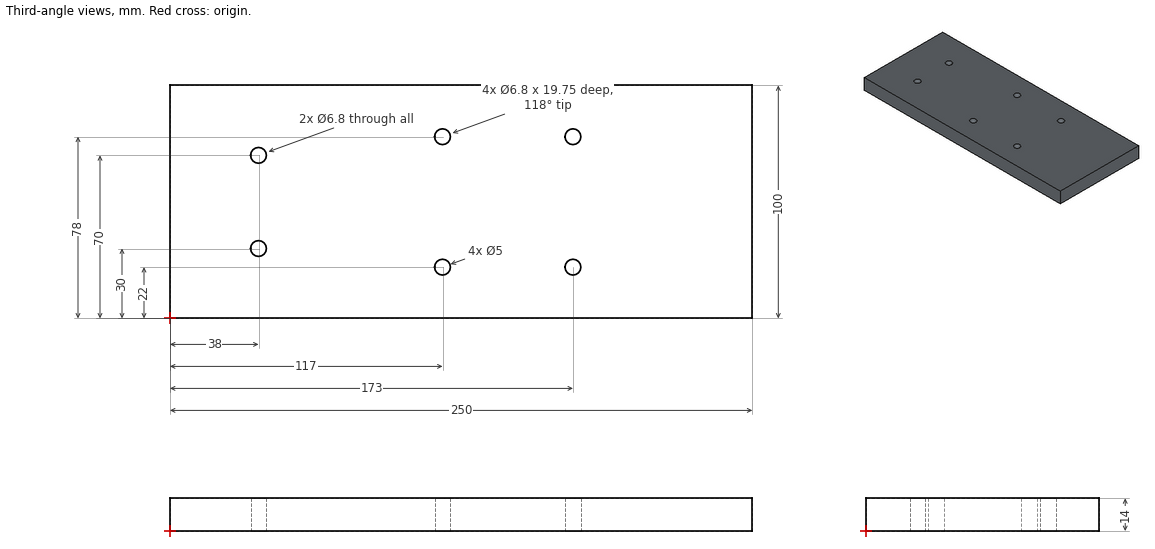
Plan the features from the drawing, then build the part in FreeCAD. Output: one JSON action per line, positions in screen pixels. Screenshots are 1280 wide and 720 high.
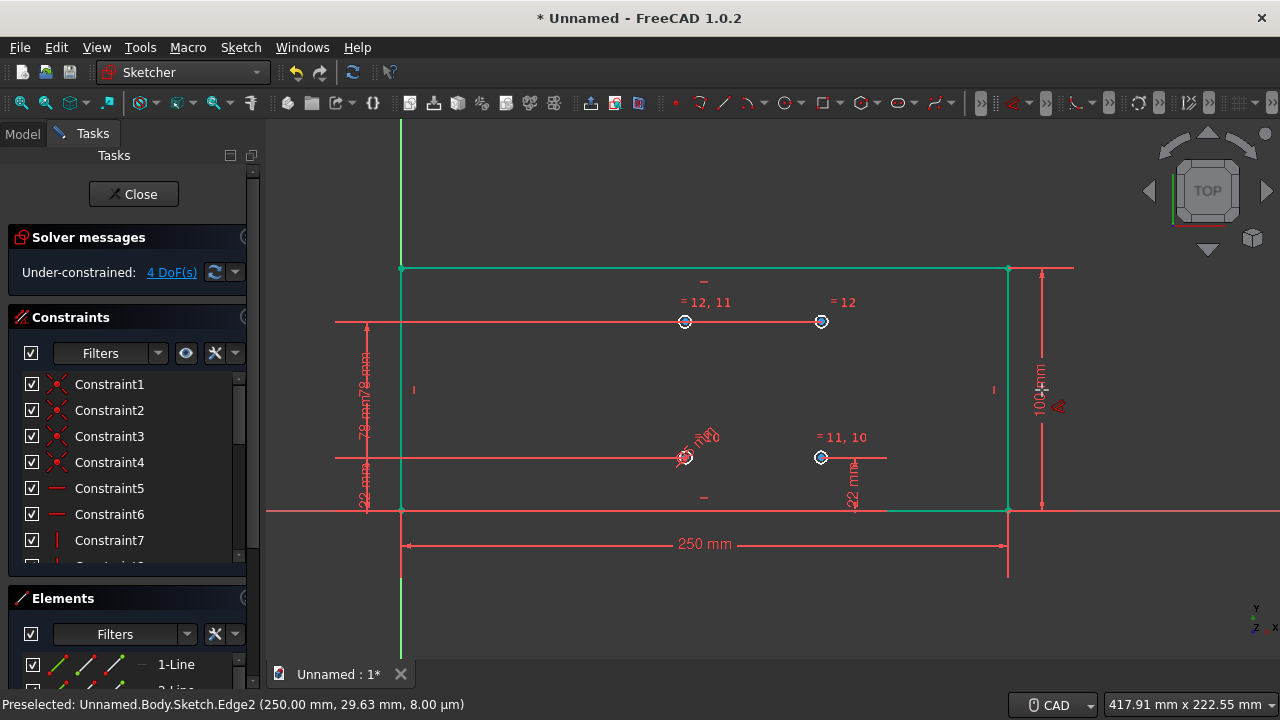
{"action": "left_click", "coordinate": [686, 458]}
{"action": "left_click", "coordinate": [544, 545]}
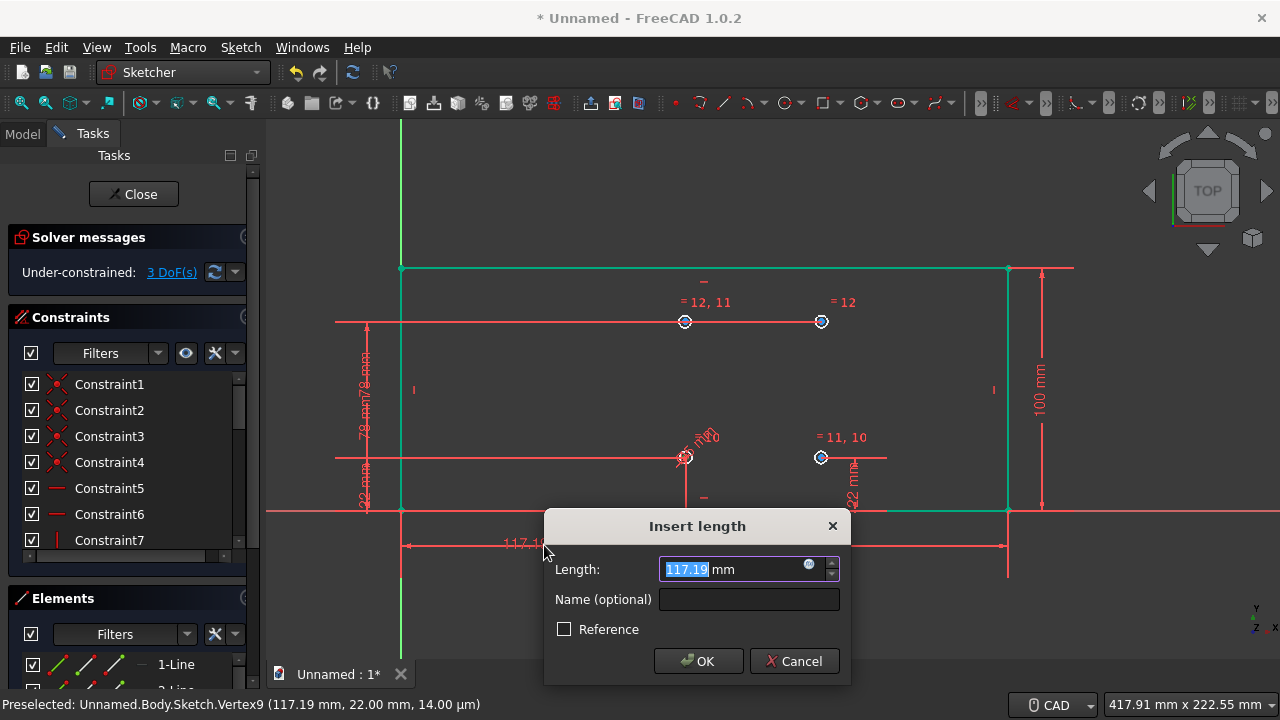
{"action": "type", "text": "117"}
{"action": "key", "text": "Return"}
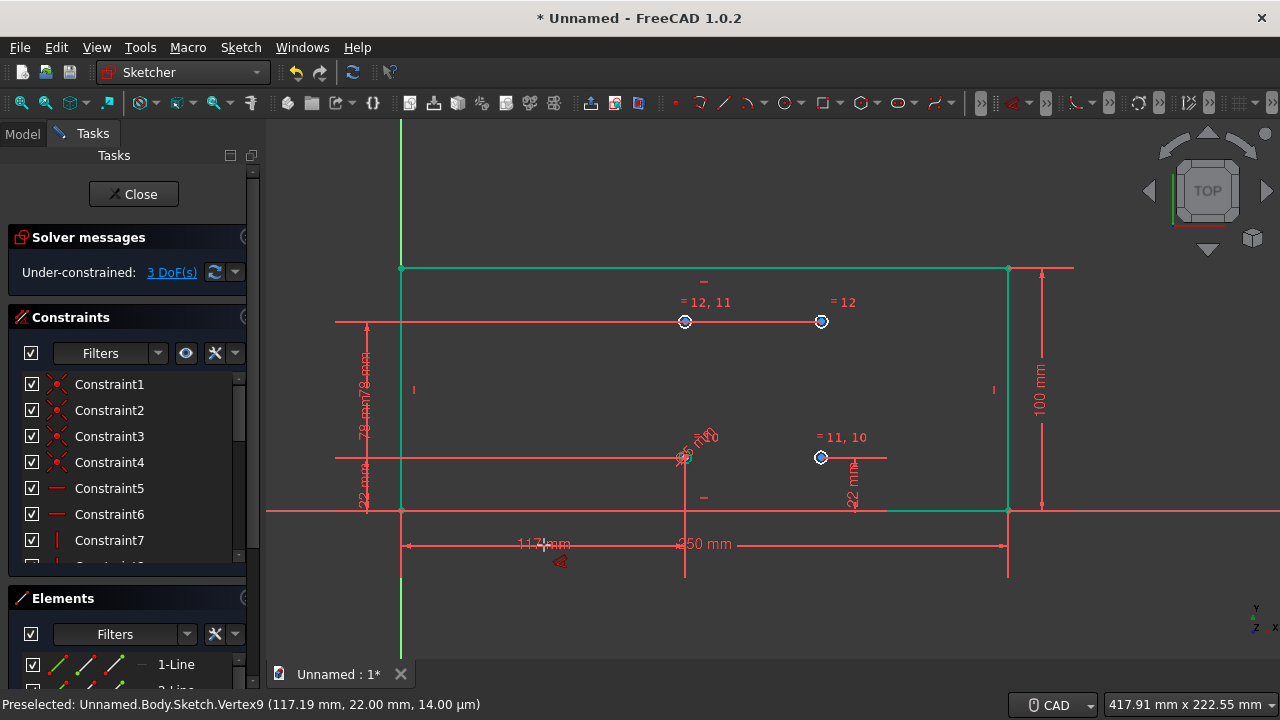
{"action": "left_click", "coordinate": [821, 458]}
{"action": "left_click", "coordinate": [464, 545]}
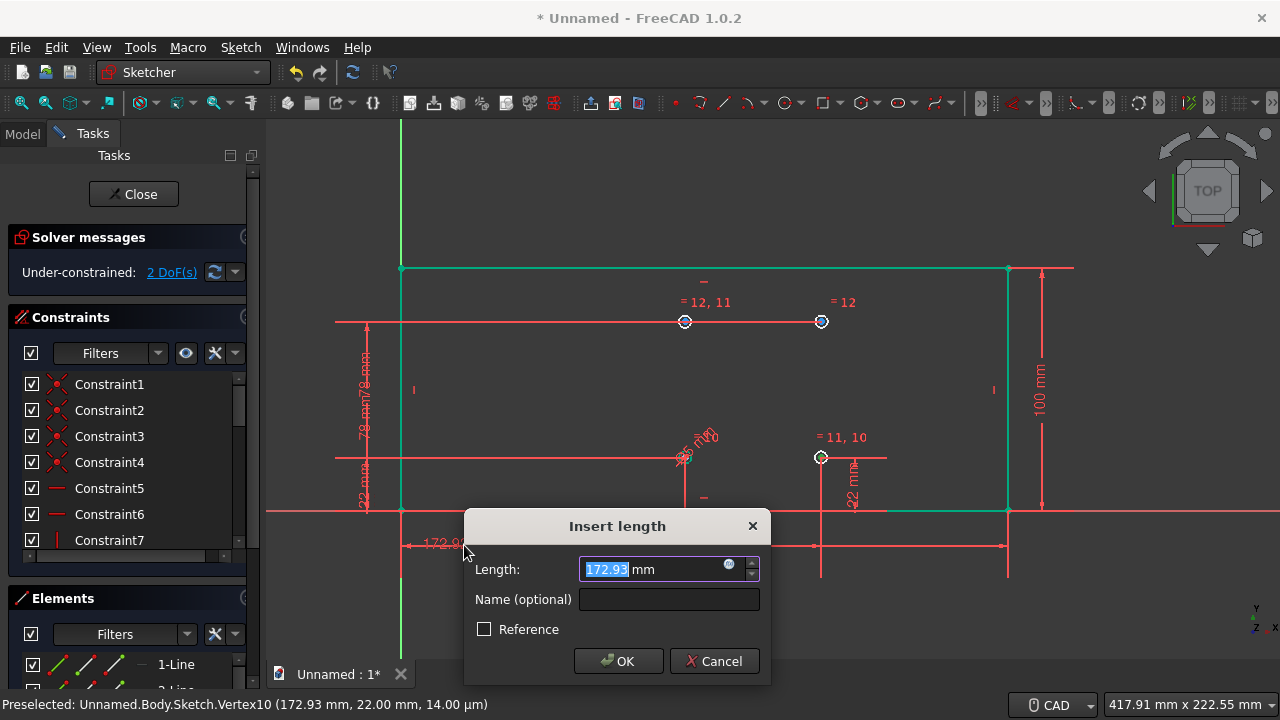
{"action": "type", "text": "173"}
{"action": "key", "text": "Return"}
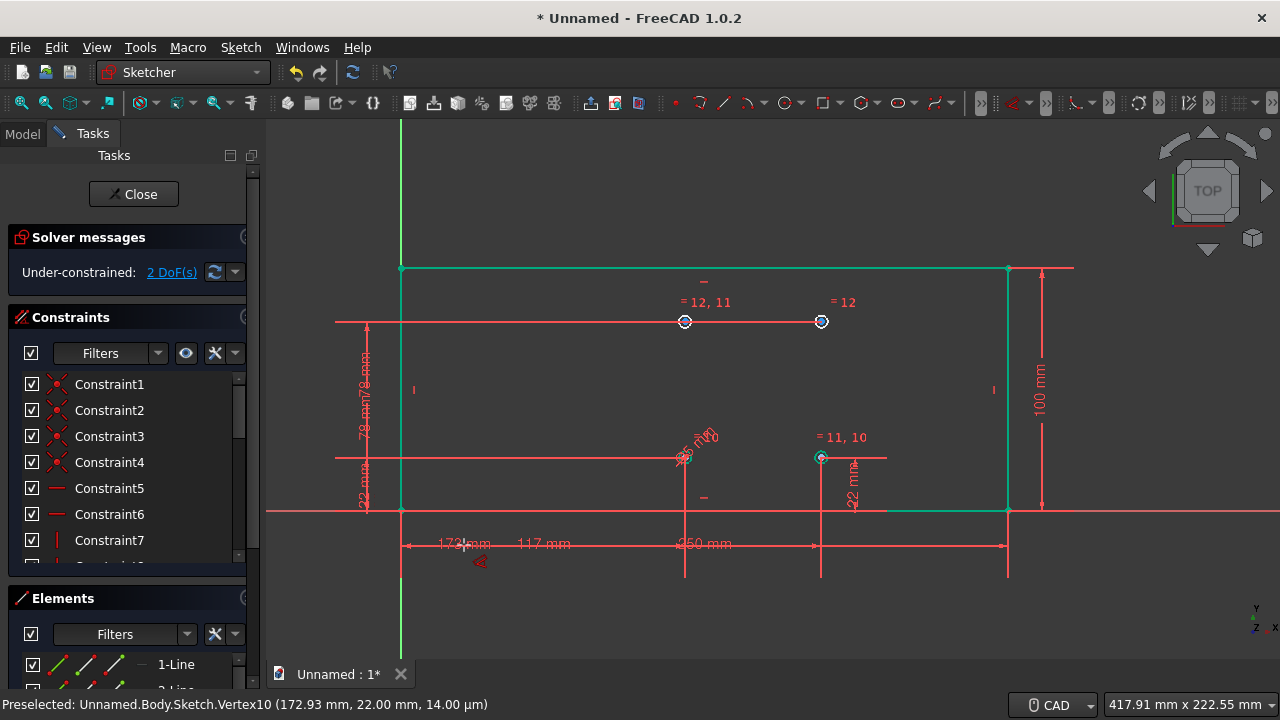
{"action": "left_click", "coordinate": [685, 322]}
{"action": "left_click", "coordinate": [543, 288]}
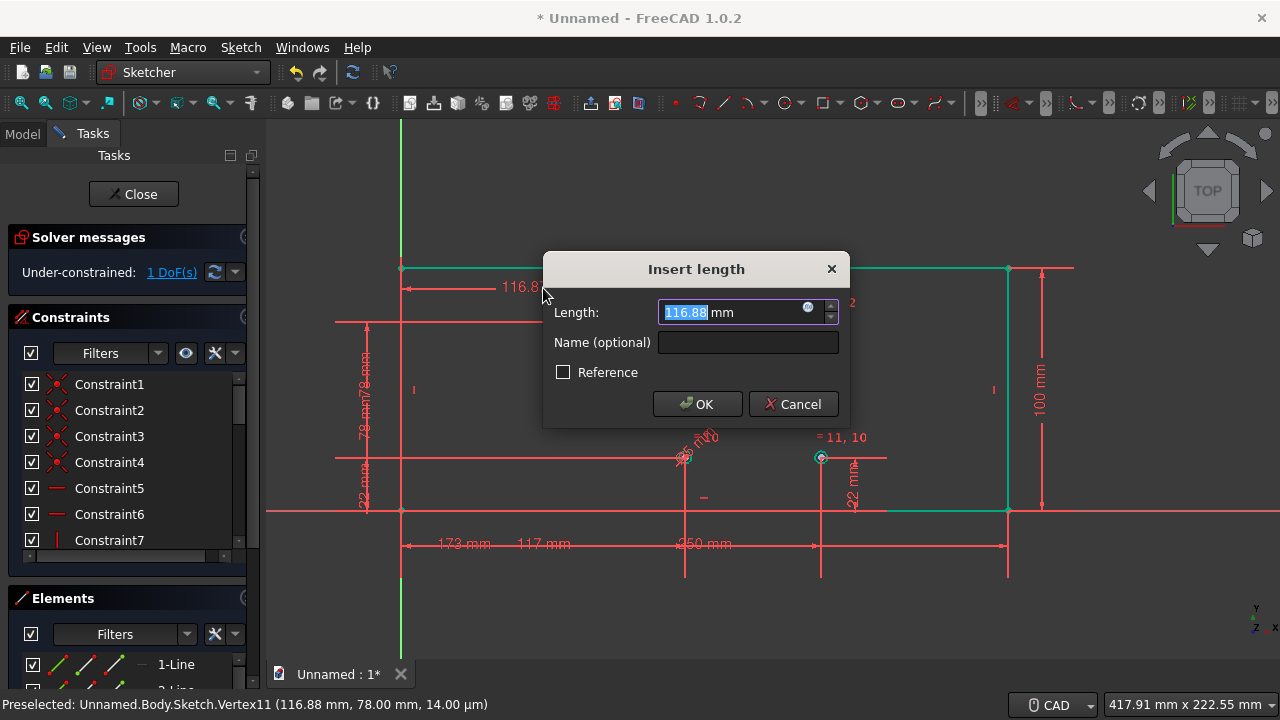
{"action": "type", "text": "117"}
{"action": "key", "text": "Return"}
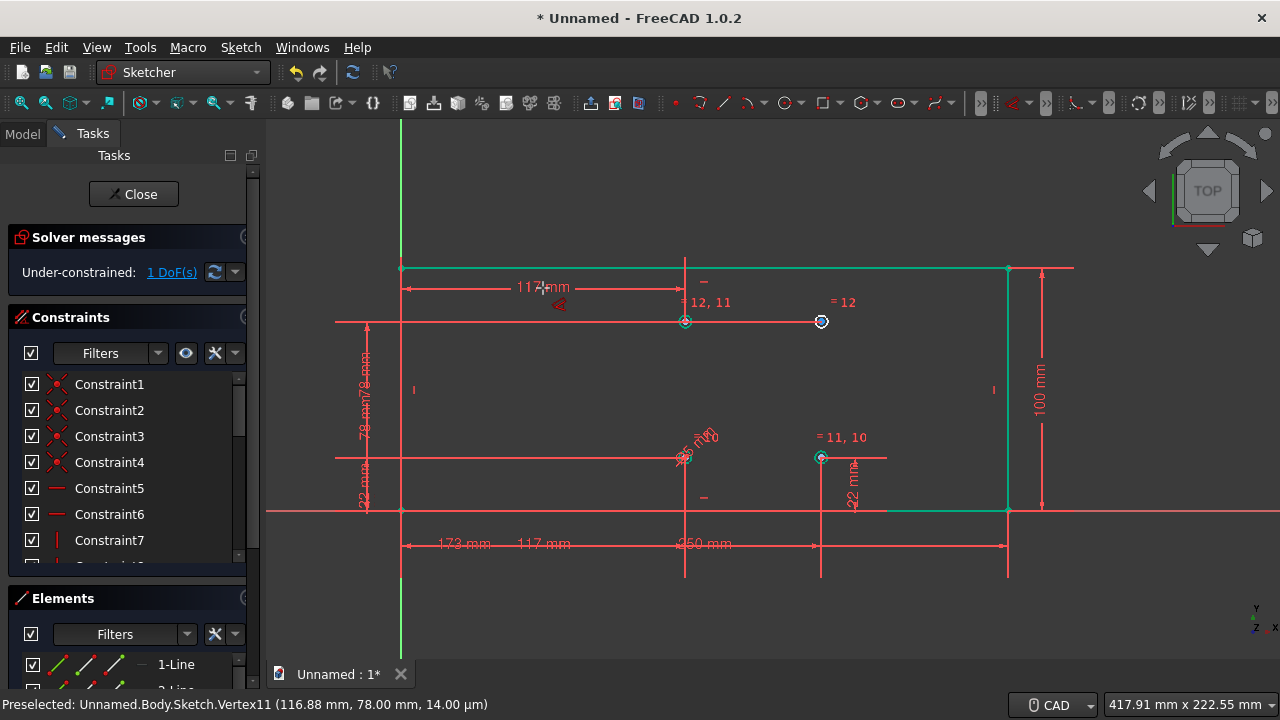
{"action": "left_click", "coordinate": [822, 322]}
{"action": "left_click", "coordinate": [708, 288]}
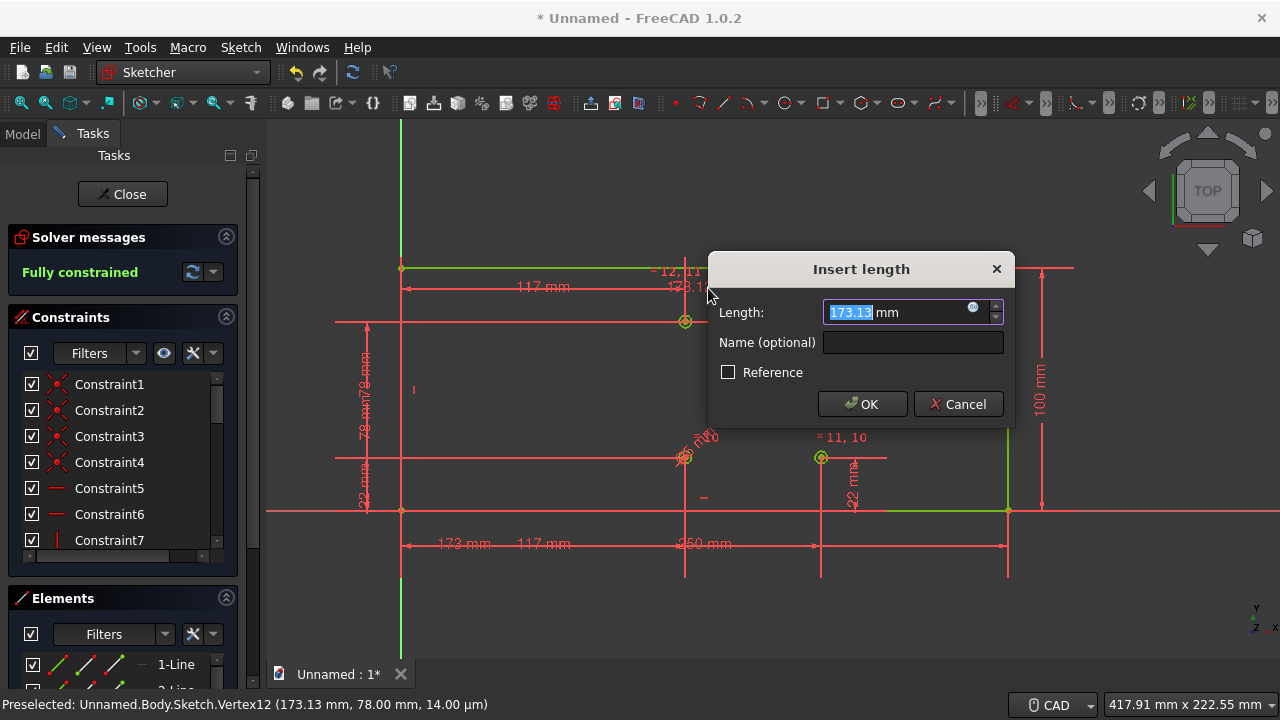
{"action": "type", "text": "173"}
{"action": "key", "text": "Return"}
{"action": "key", "text": "Escape"}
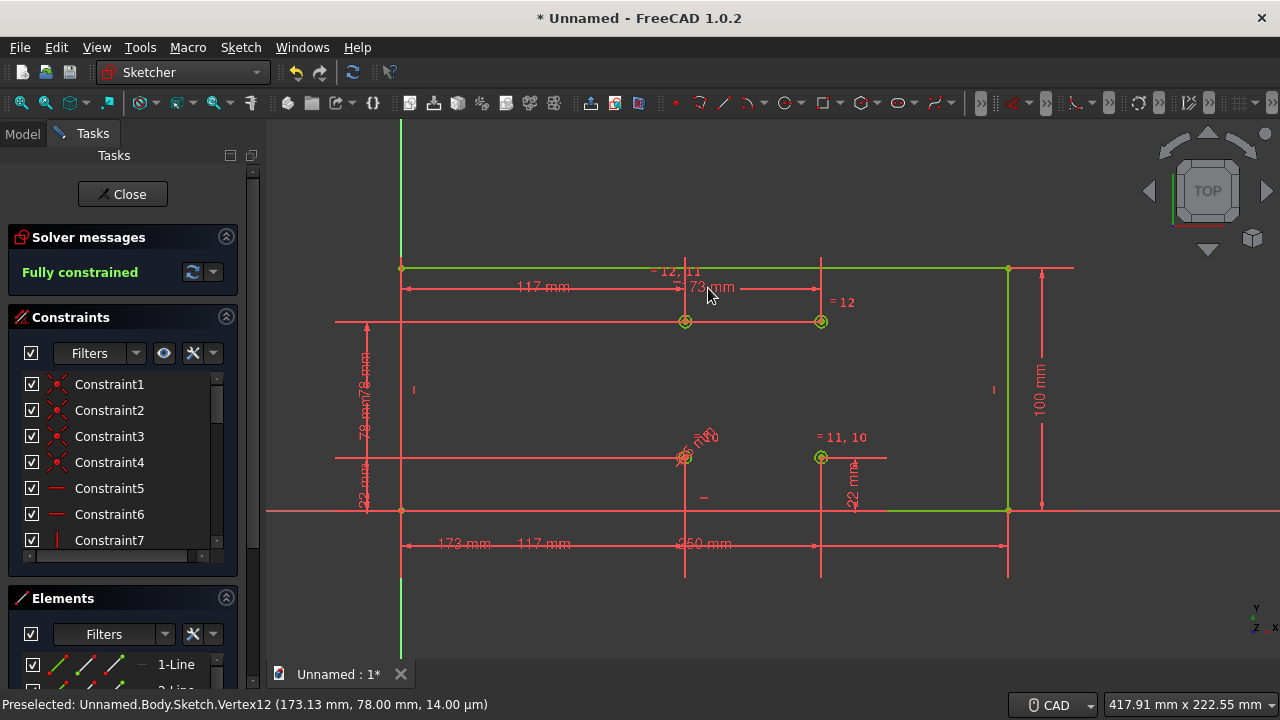
{"action": "left_click", "coordinate": [123, 194]}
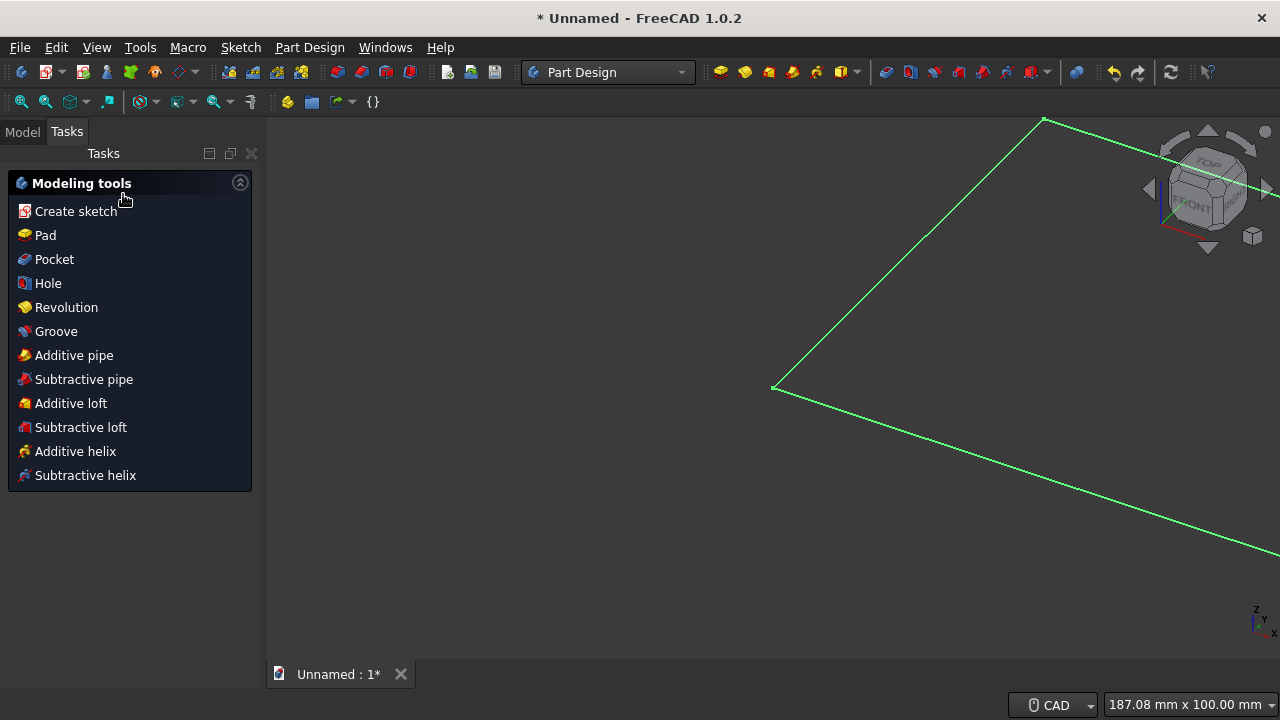
{"action": "left_click", "coordinate": [722, 72]}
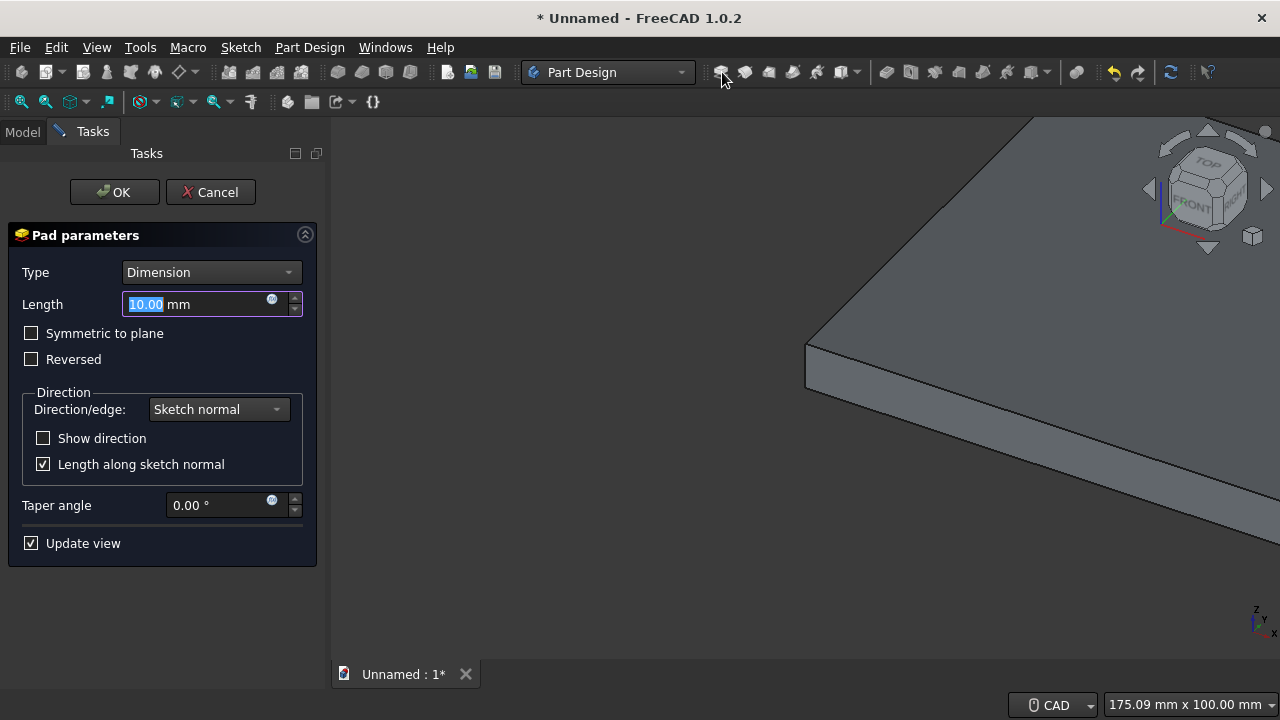
{"action": "type", "text": "14"}
{"action": "key", "text": "Tab"}